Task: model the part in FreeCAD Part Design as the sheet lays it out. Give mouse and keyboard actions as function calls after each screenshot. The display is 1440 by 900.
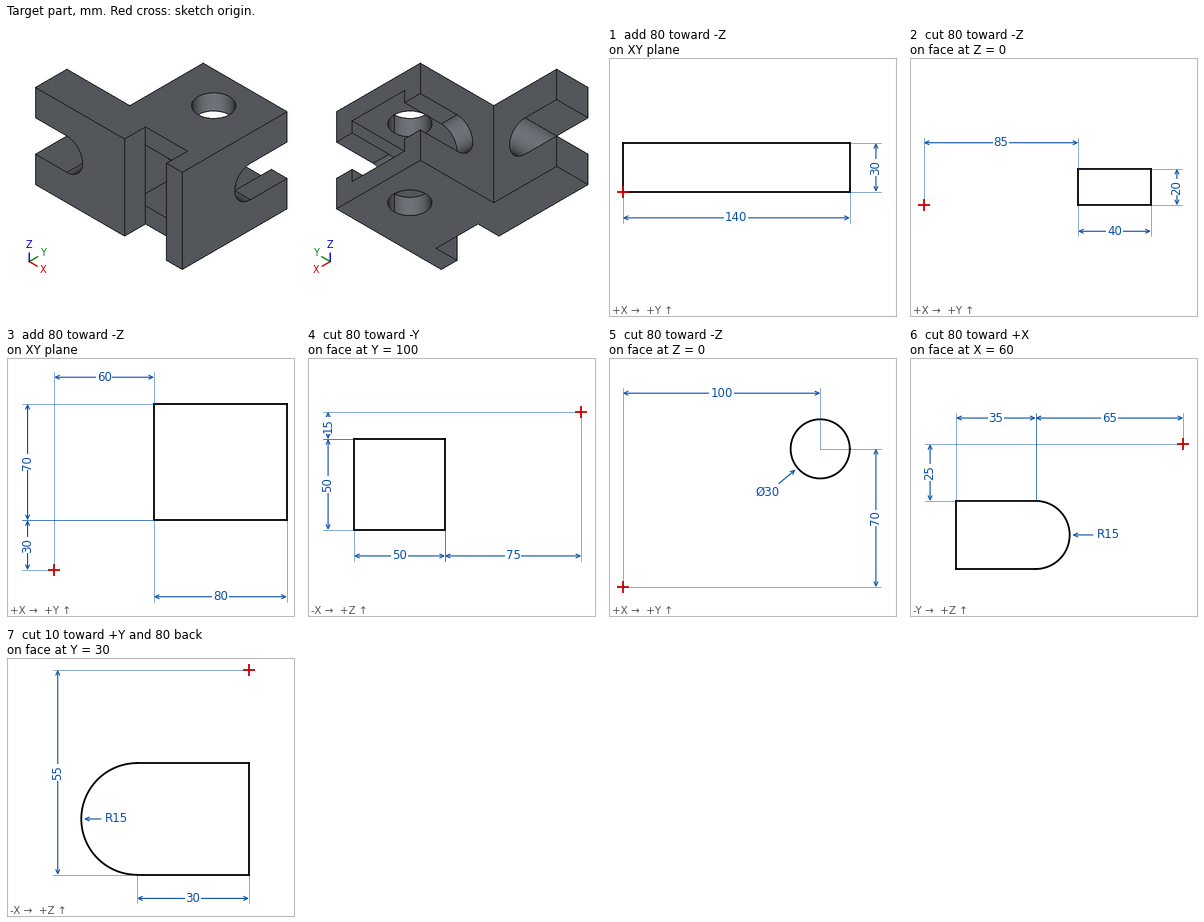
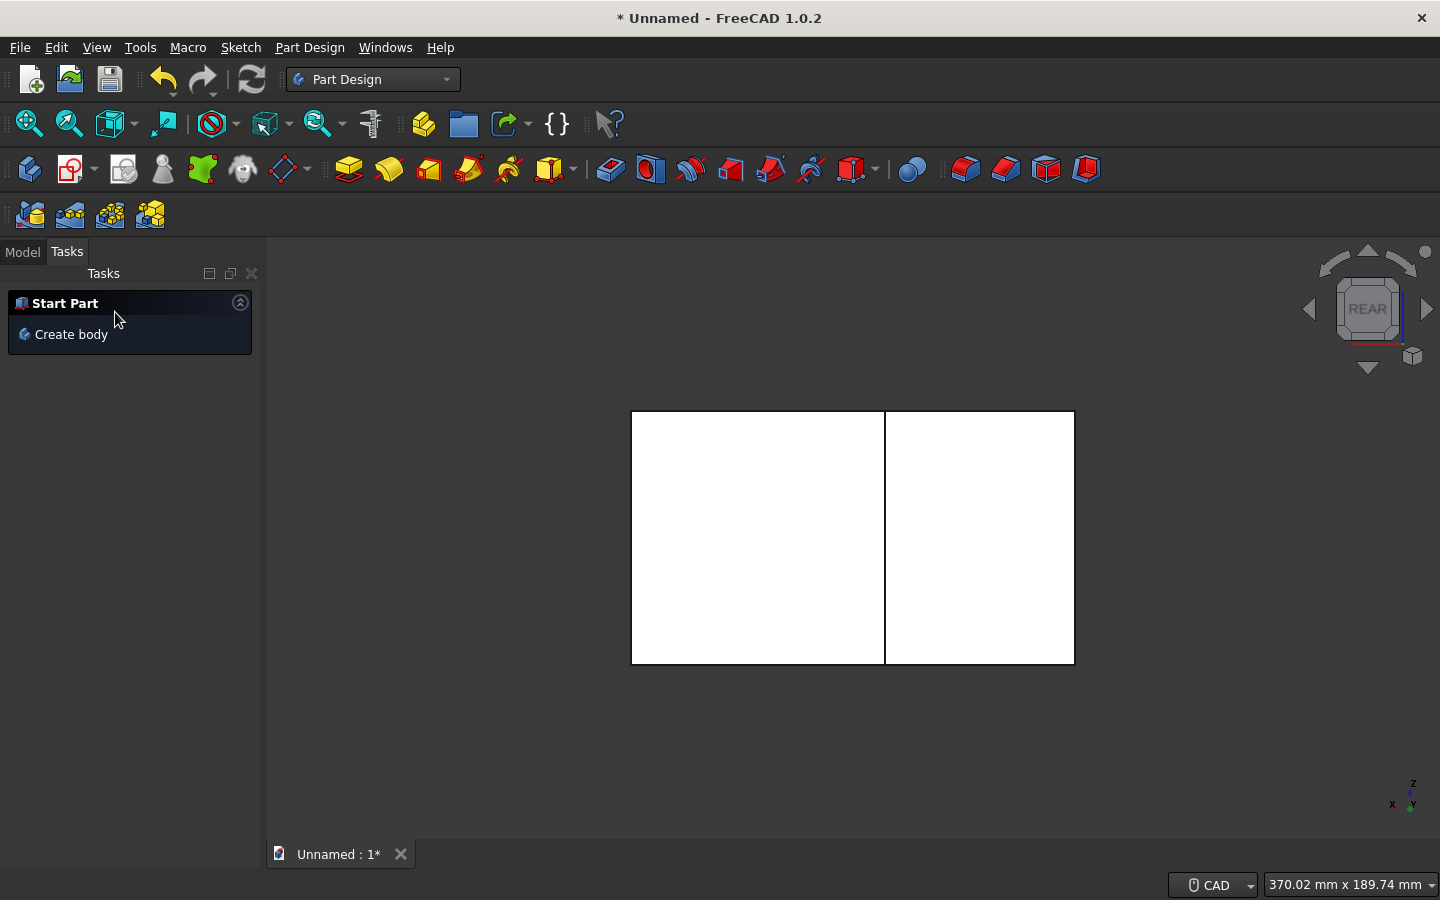
click(30, 124)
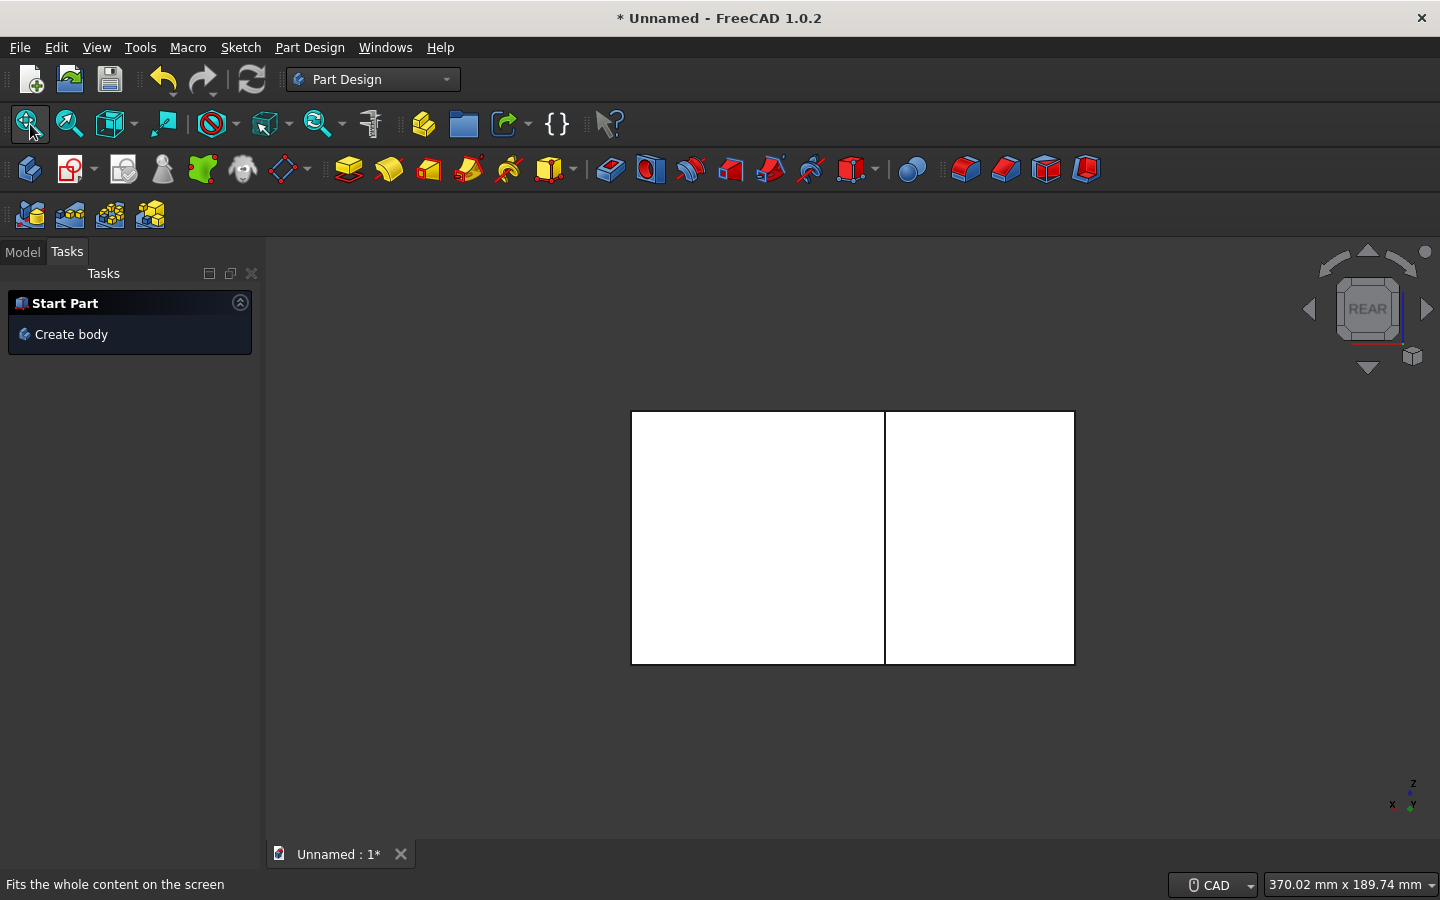
click(758, 537)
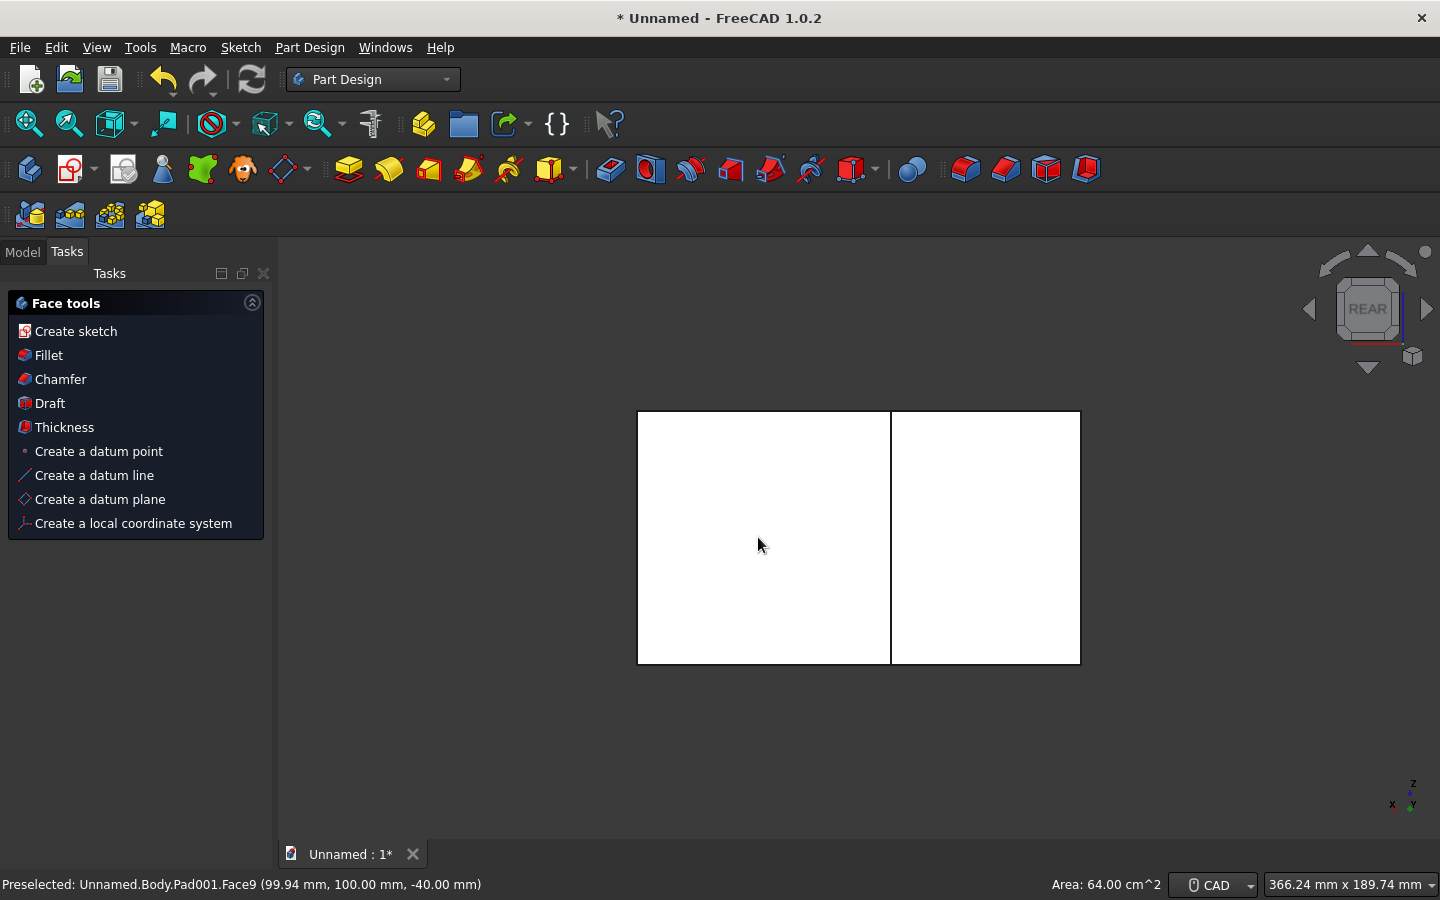
click(70, 170)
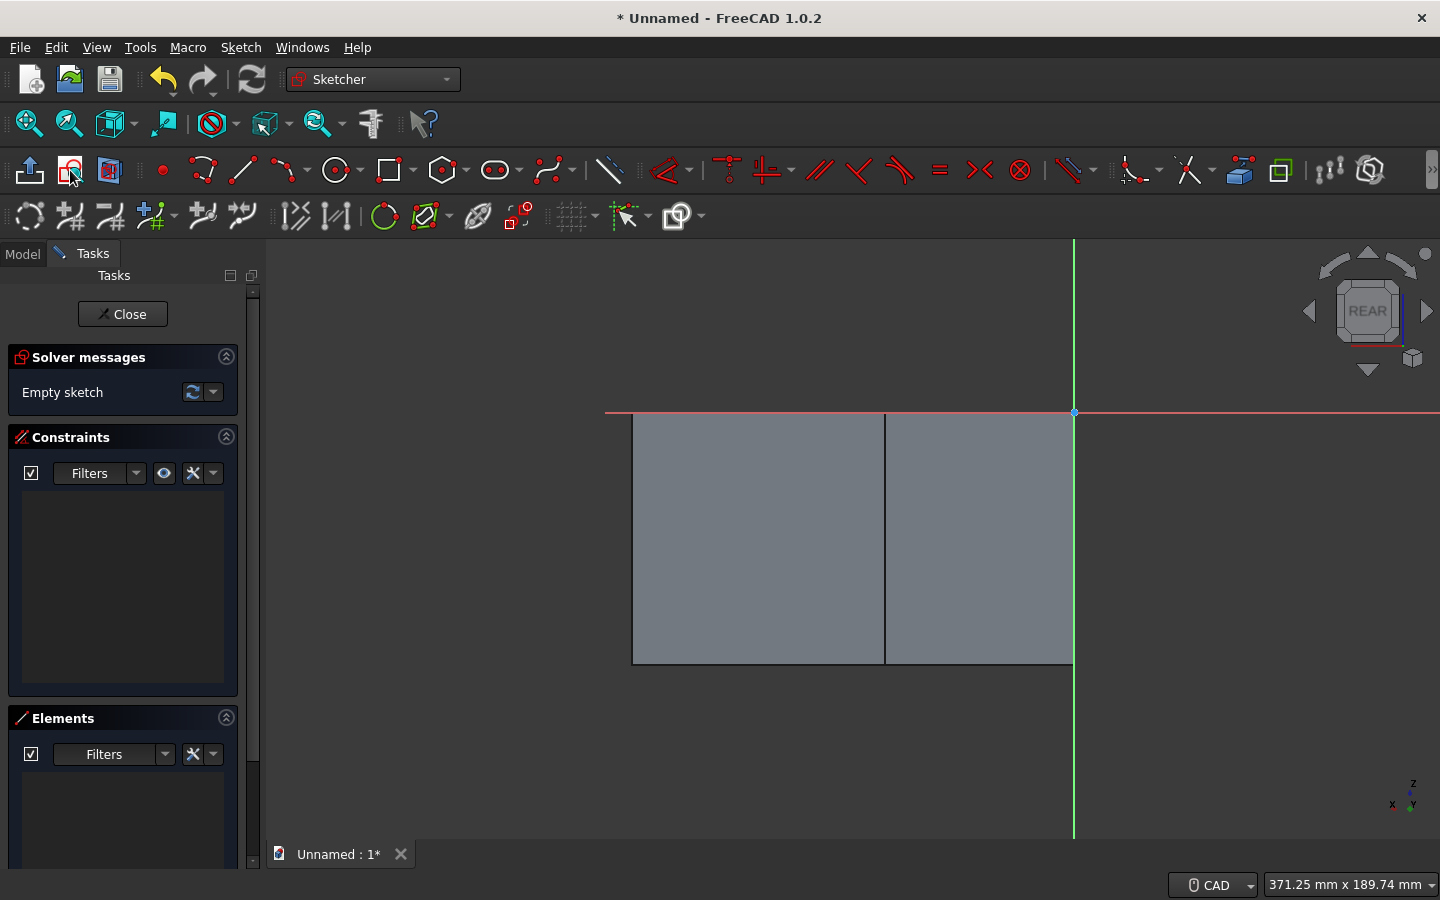
scroll(737, 539, up, 4)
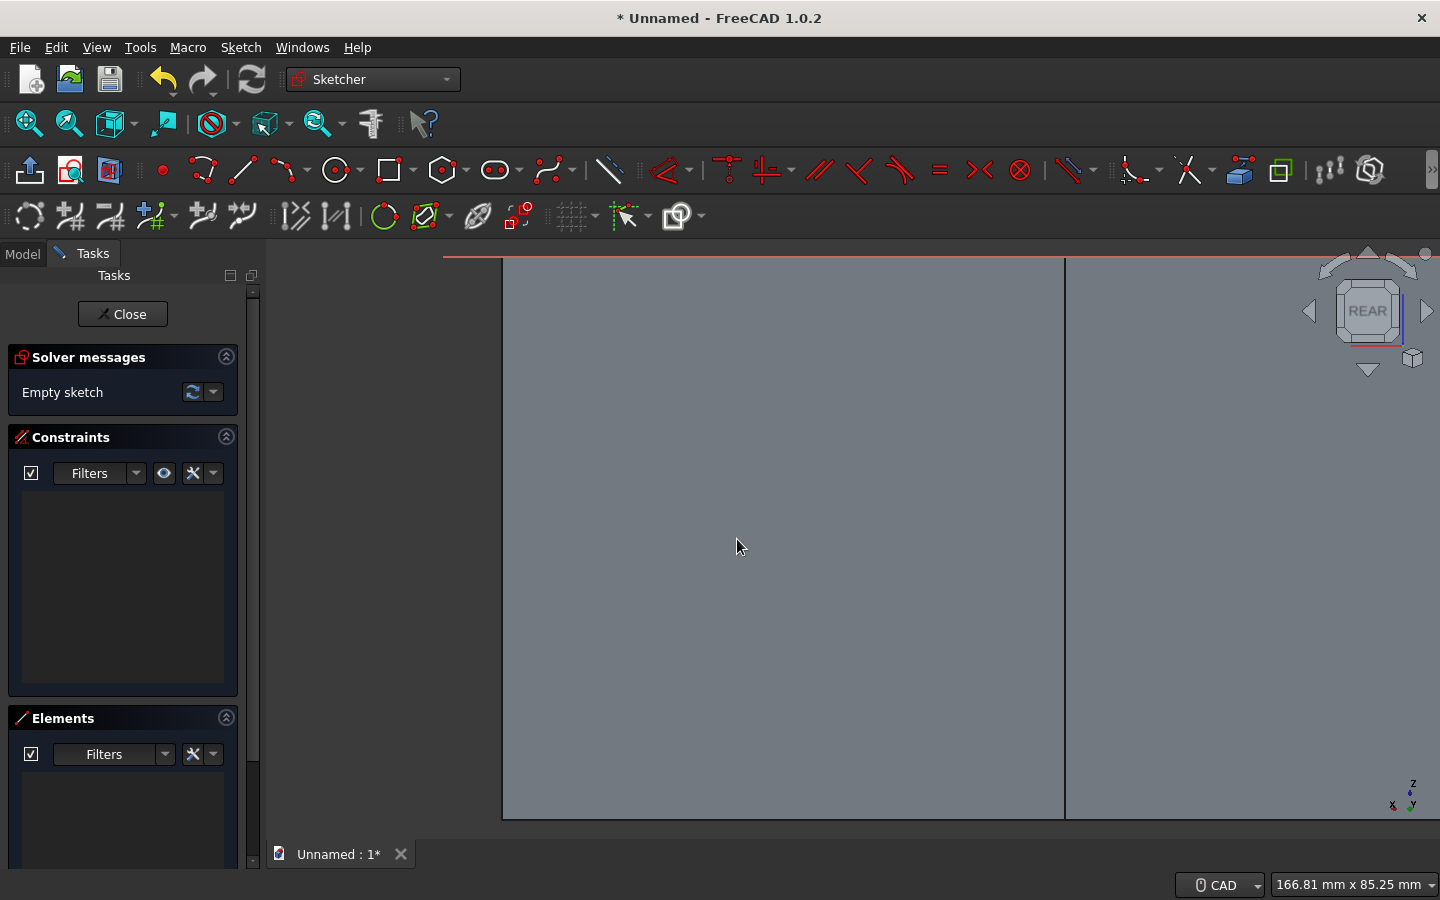
key(g)
key(r)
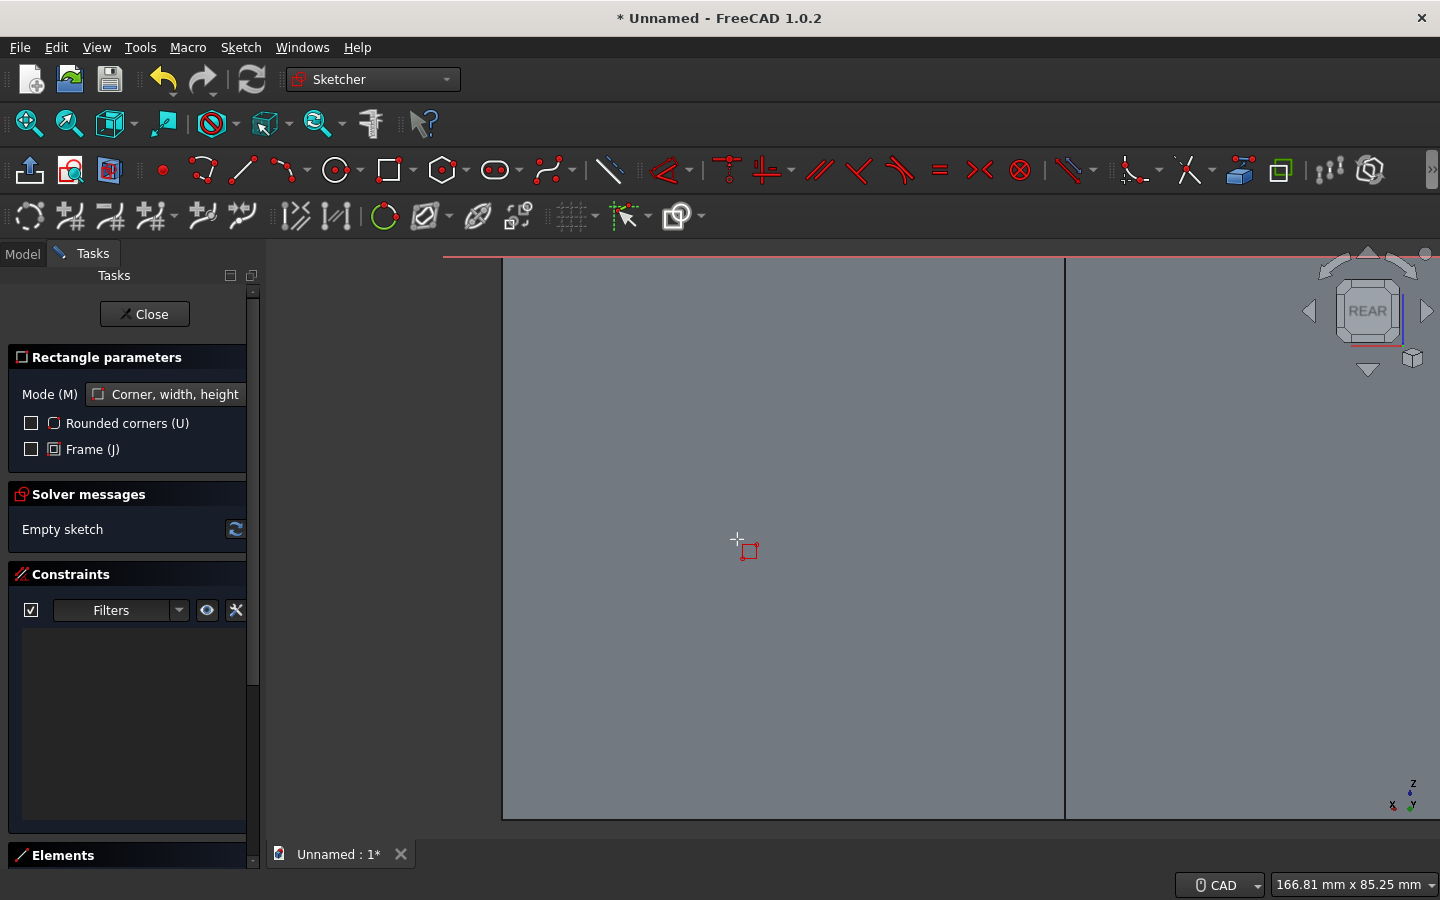
click(608, 362)
click(959, 714)
key(Escape)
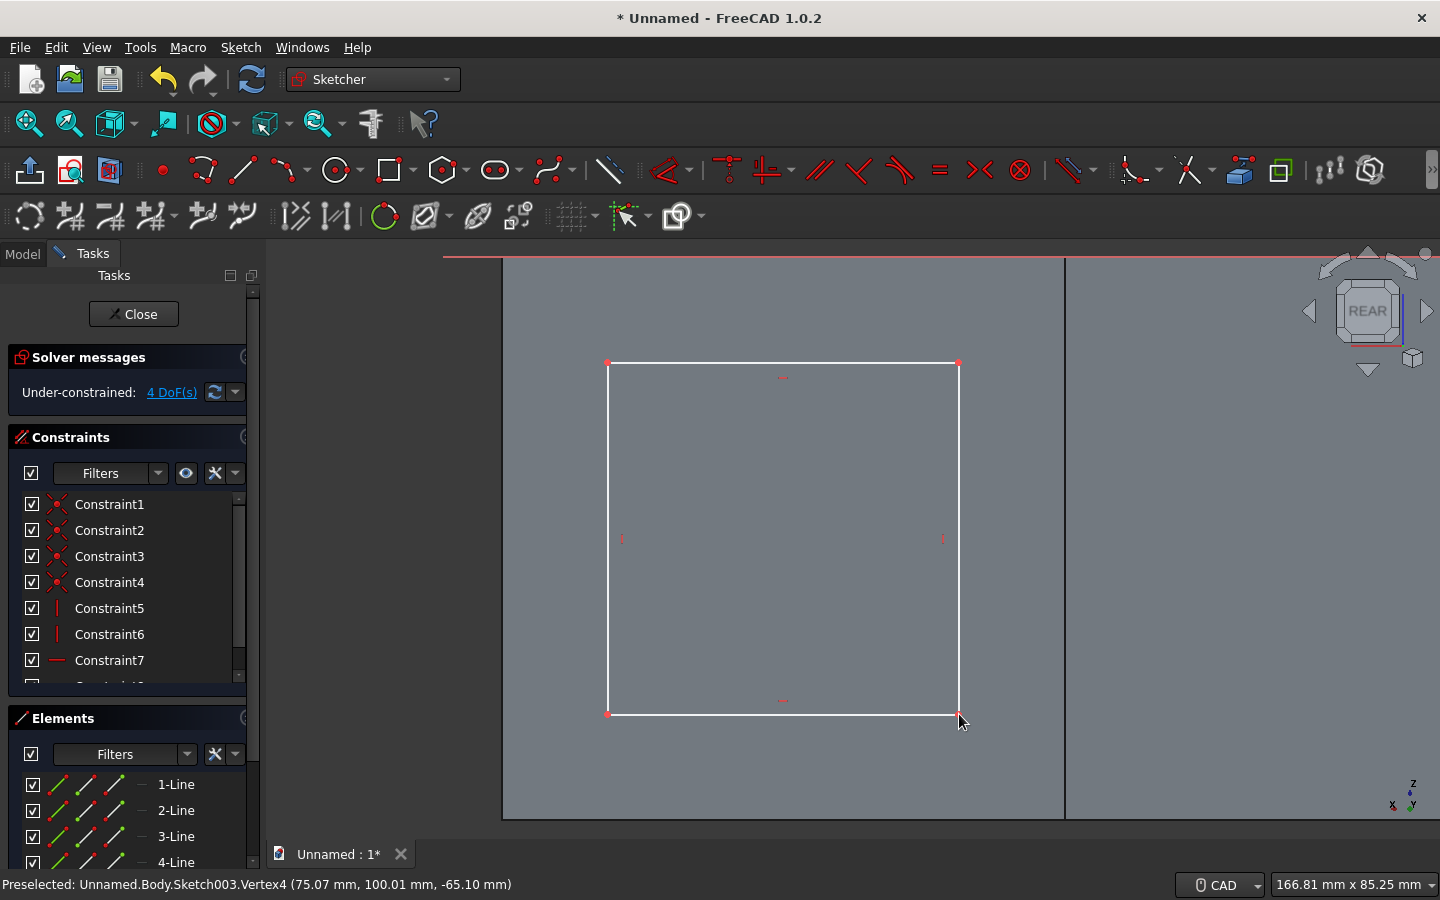
key(d)